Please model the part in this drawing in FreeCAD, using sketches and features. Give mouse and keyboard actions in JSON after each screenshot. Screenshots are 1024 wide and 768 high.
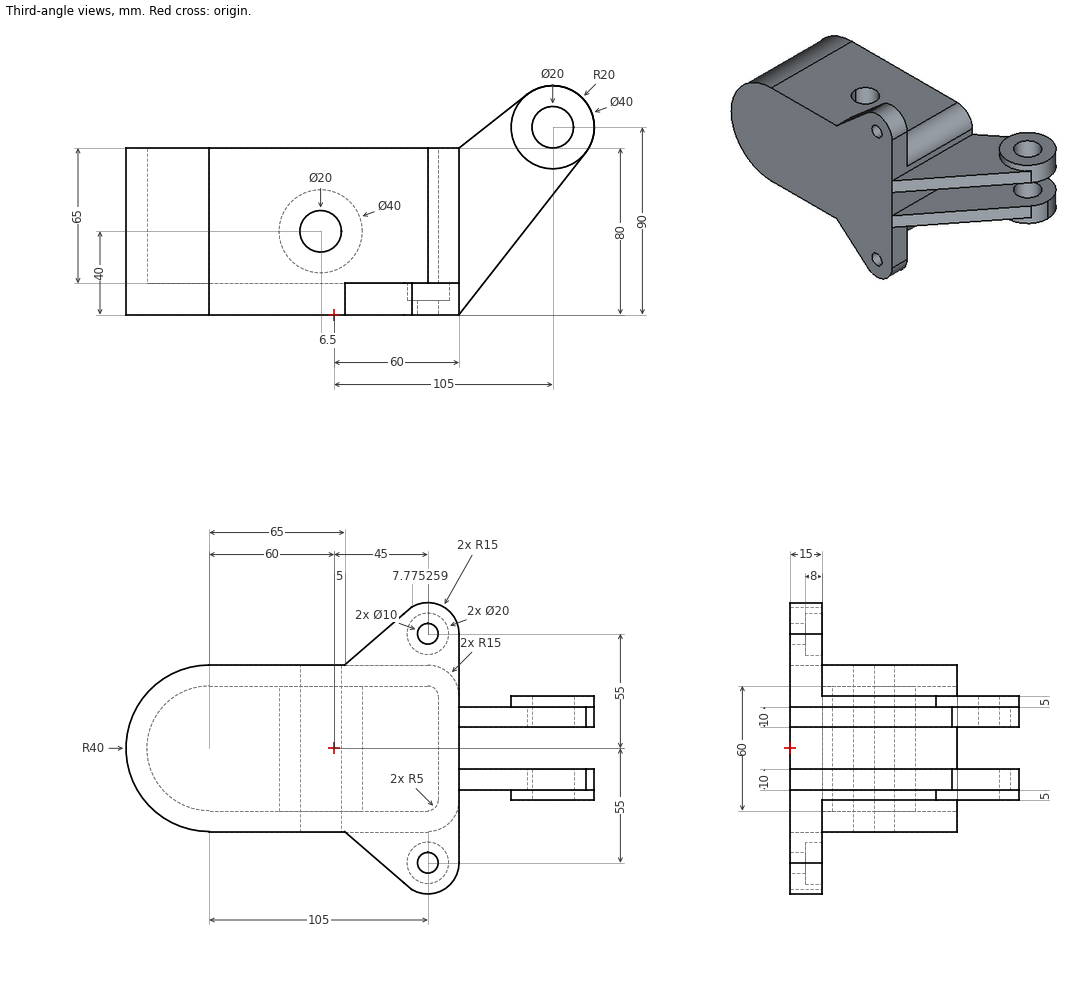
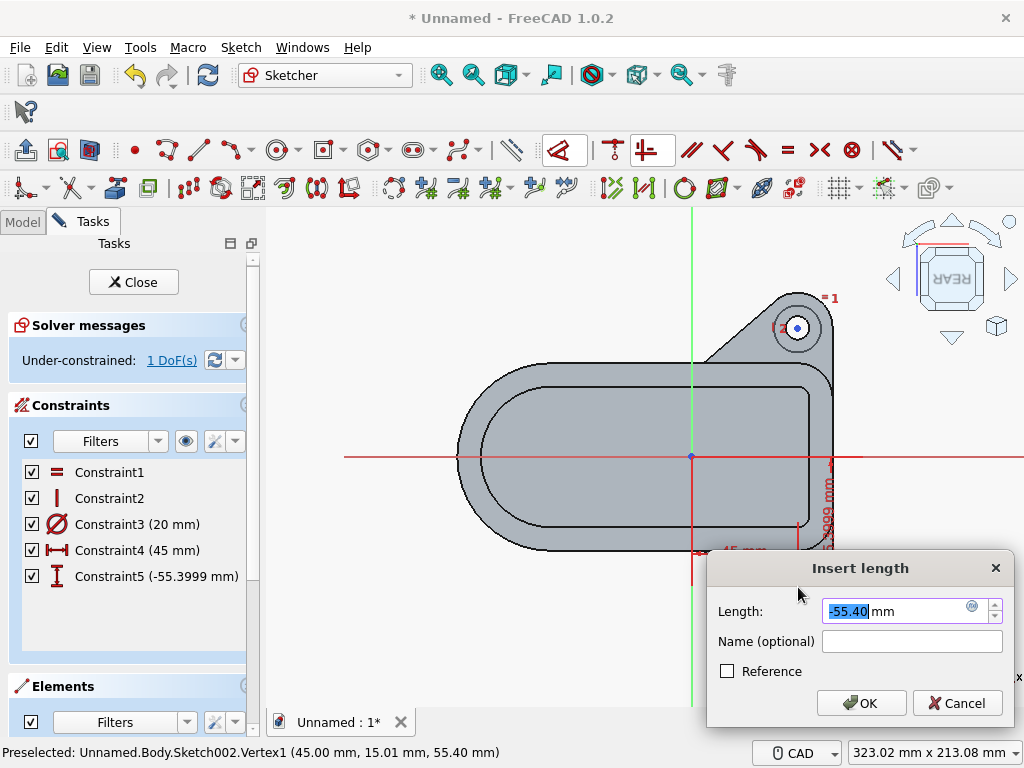
{"action": "type", "text": "-55"}
{"action": "key", "text": "Return"}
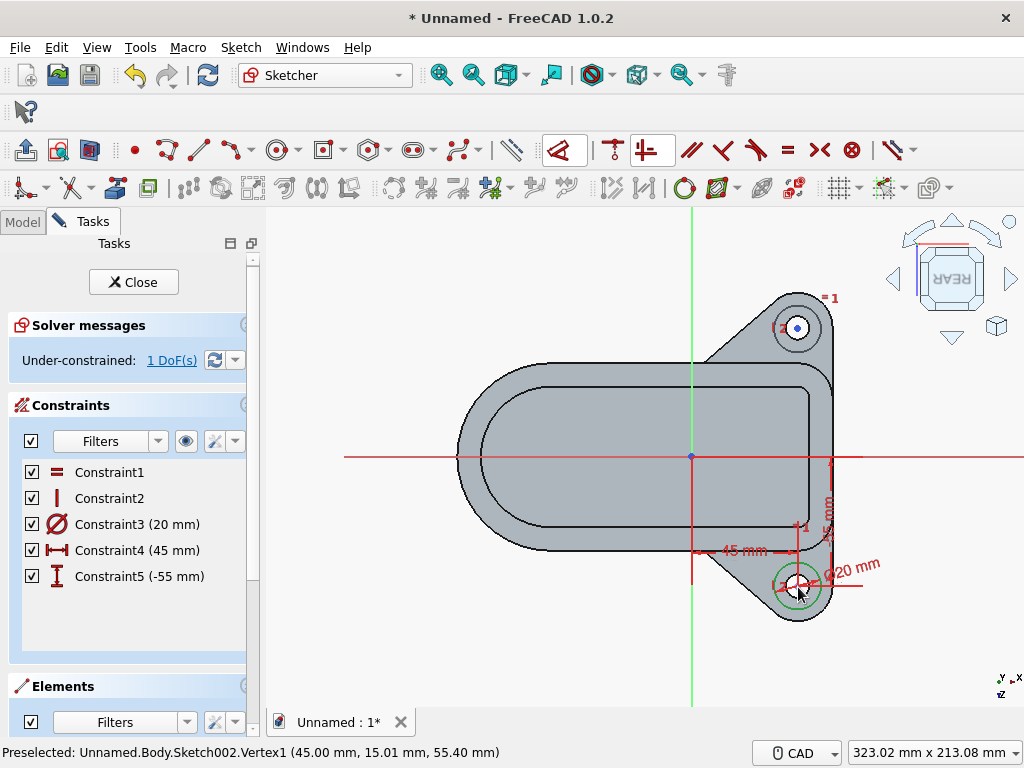
{"action": "left_click", "coordinate": [798, 329]}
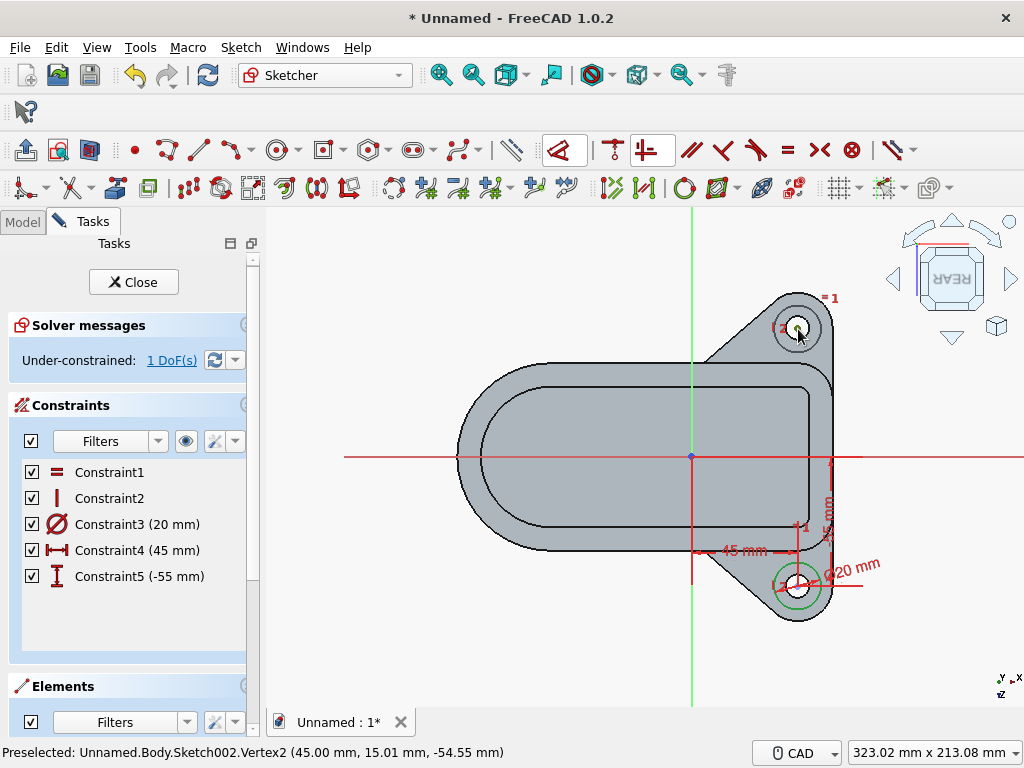
{"action": "key", "text": "i"}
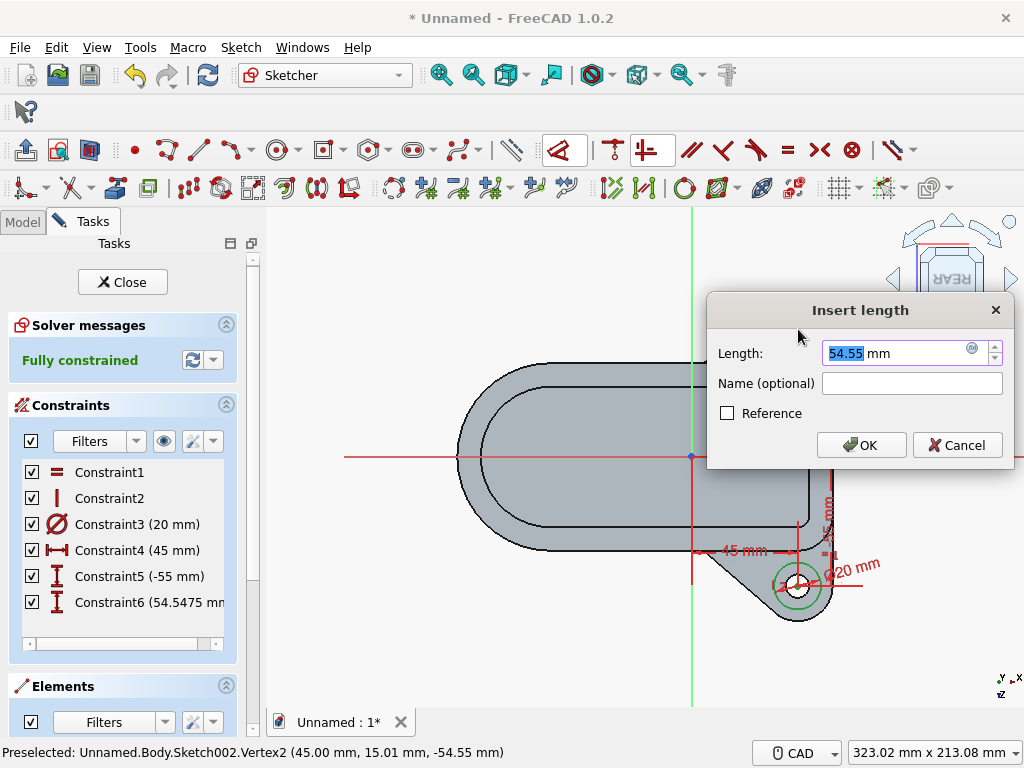
{"action": "type", "text": "55"}
{"action": "key", "text": "Return"}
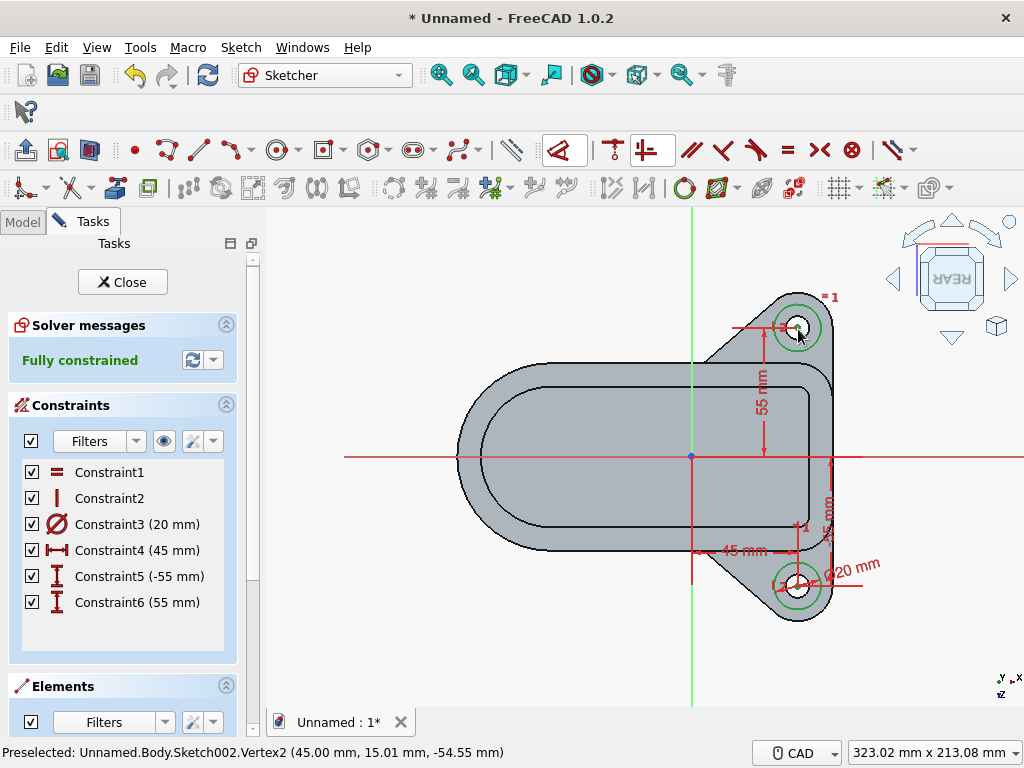
{"action": "left_click", "coordinate": [123, 282]}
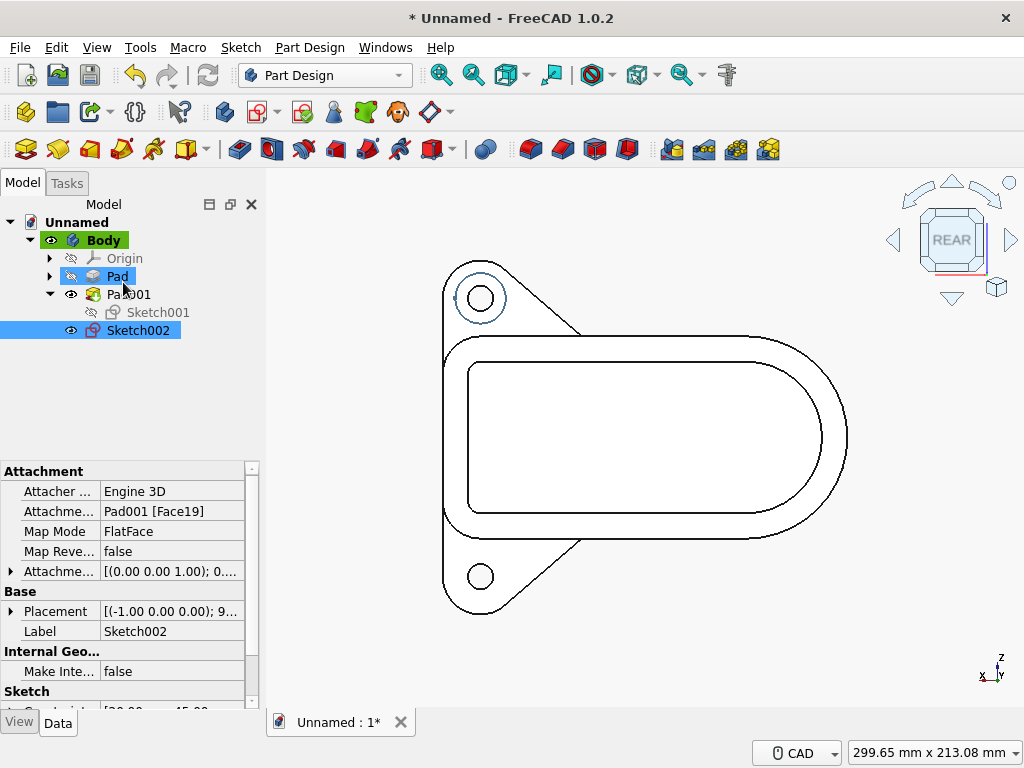
{"action": "left_click", "coordinate": [240, 150]}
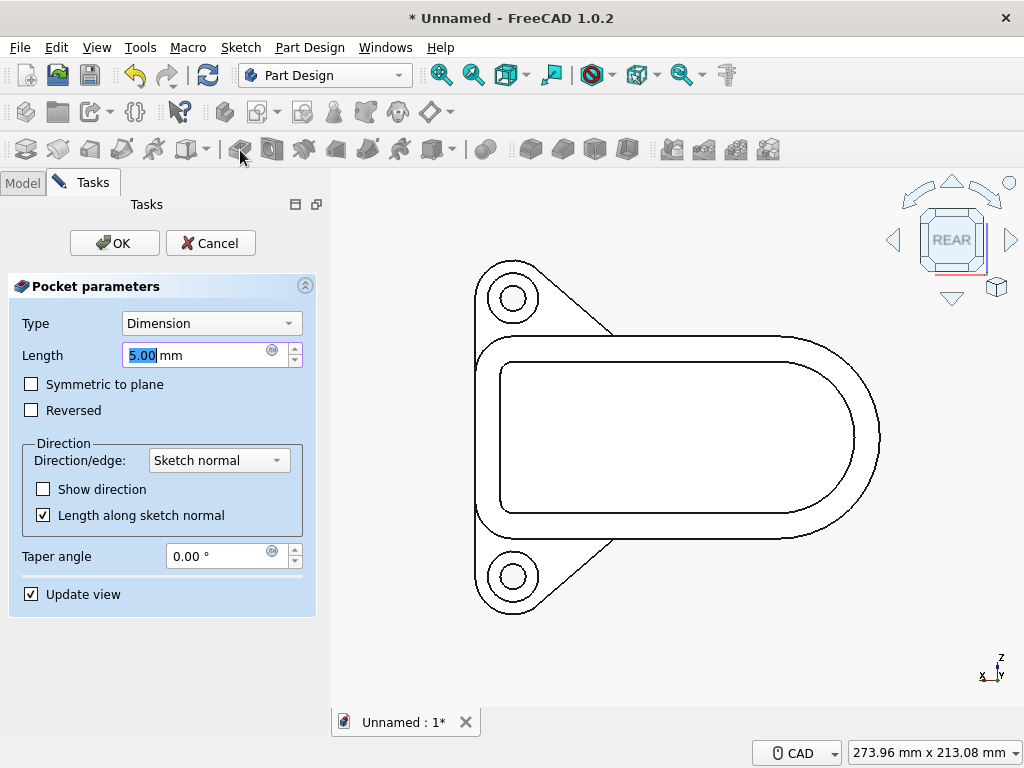
{"action": "type", "text": "8"}
{"action": "key", "text": "Tab"}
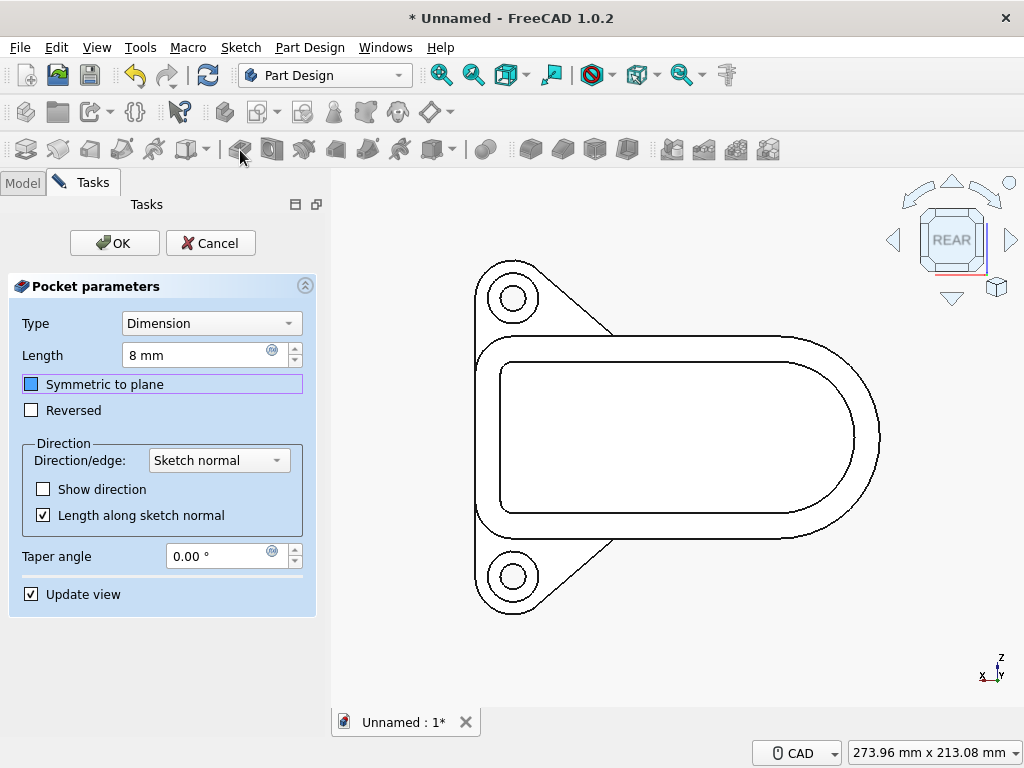
{"action": "left_click", "coordinate": [115, 243]}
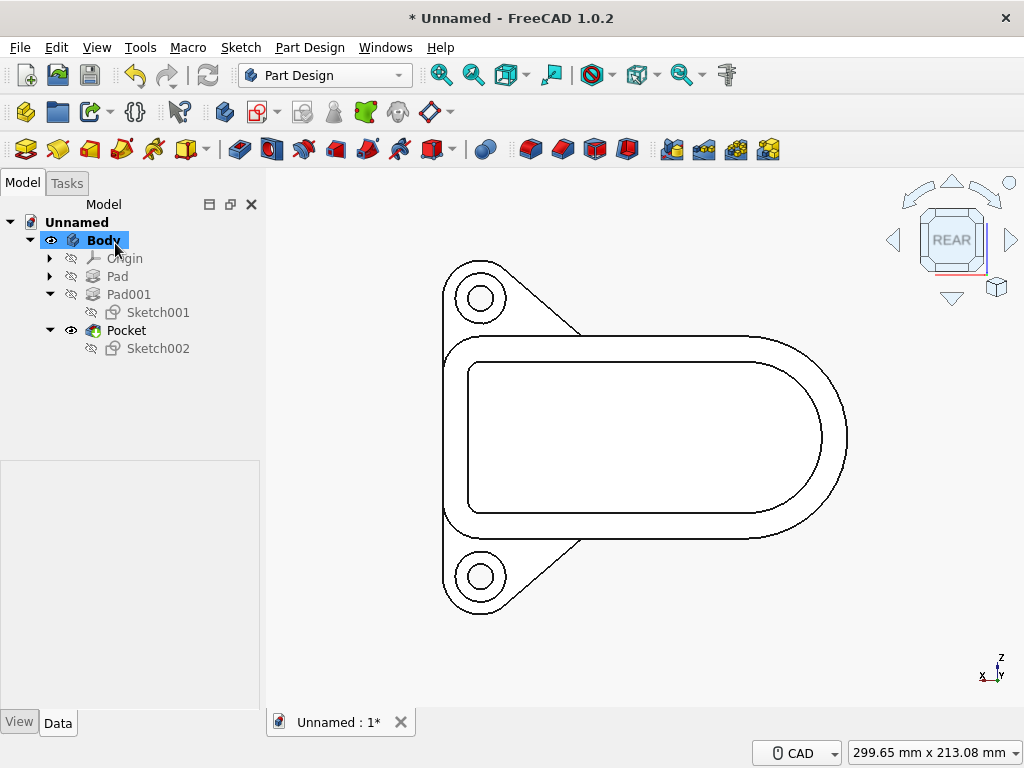
{"action": "key", "text": "0"}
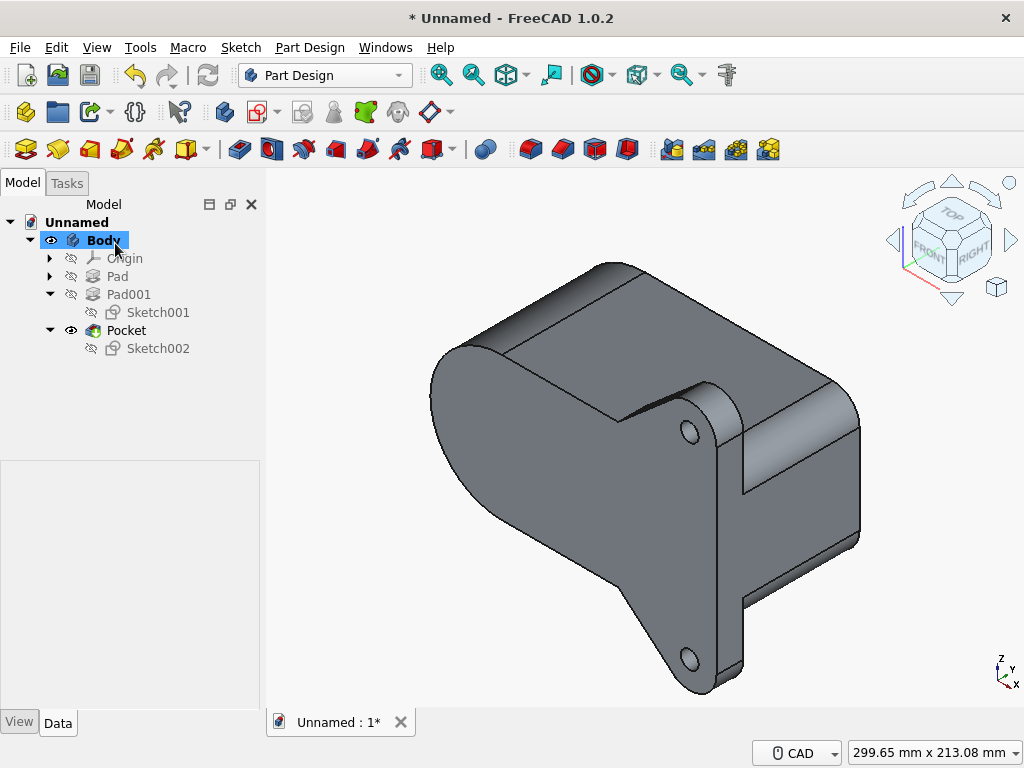
{"action": "left_click", "coordinate": [641, 351]}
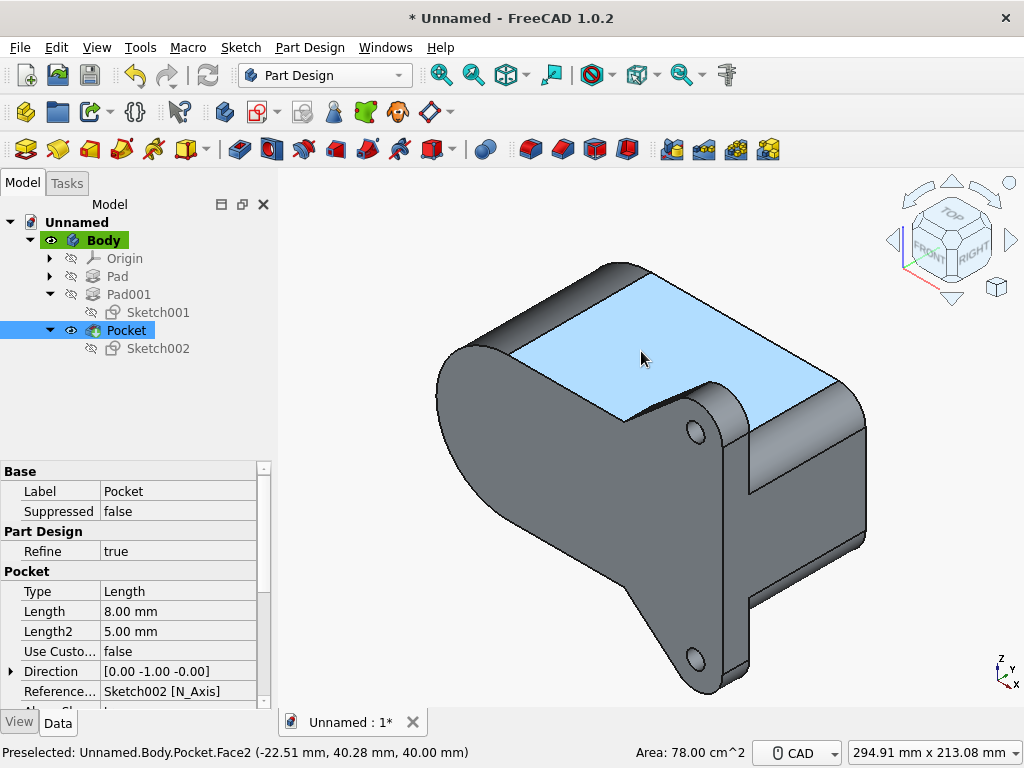
{"action": "left_click", "coordinate": [258, 112]}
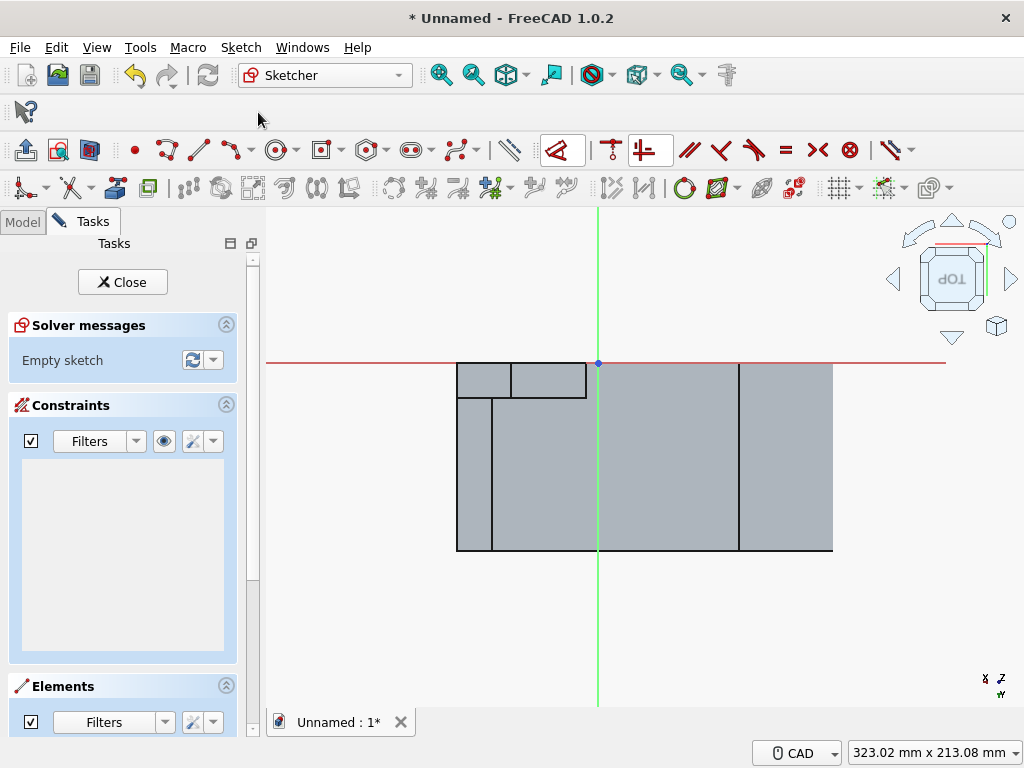
{"action": "scroll", "coordinate": [621, 457], "scroll_direction": "up", "scroll_amount": 9}